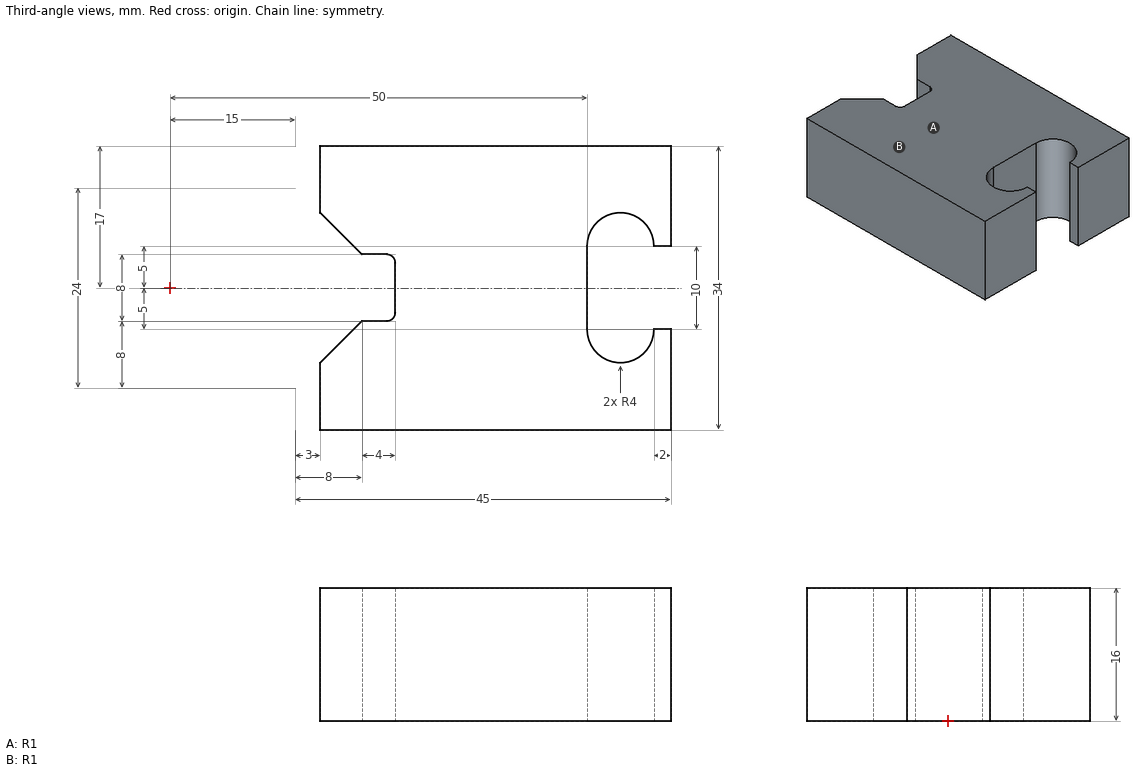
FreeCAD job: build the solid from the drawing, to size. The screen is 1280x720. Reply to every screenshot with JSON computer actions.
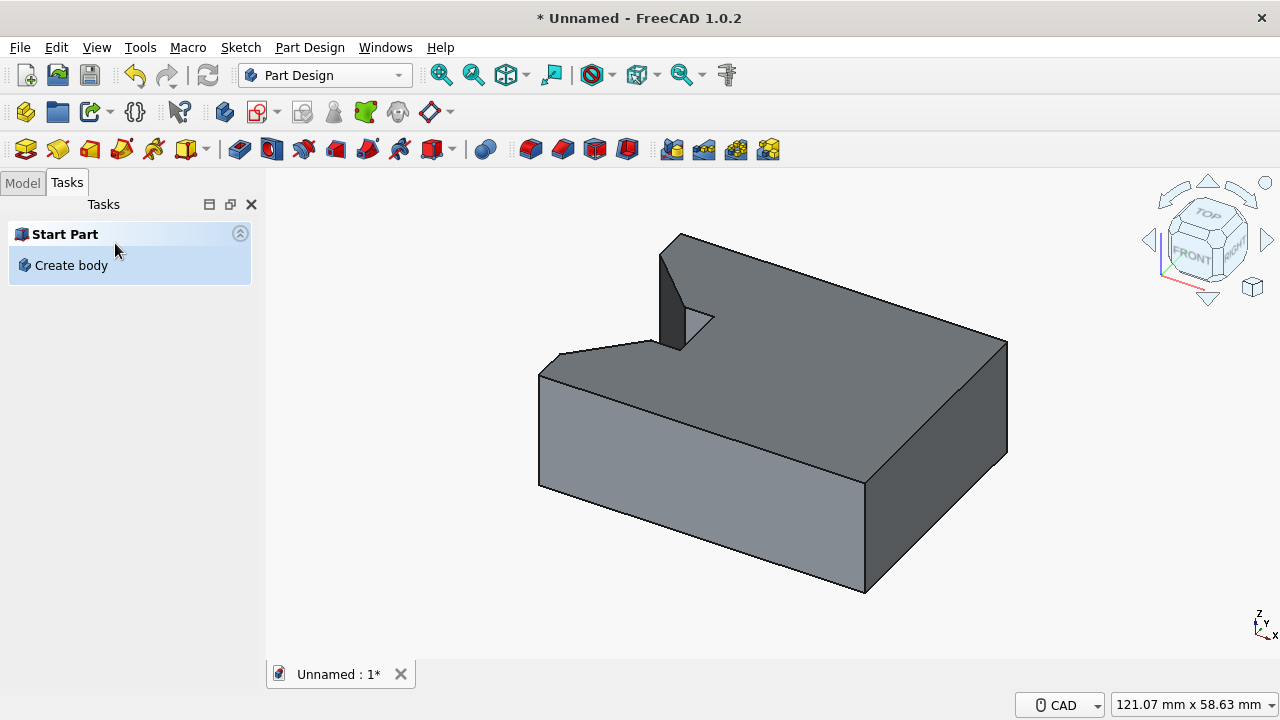
{"action": "key", "text": "0"}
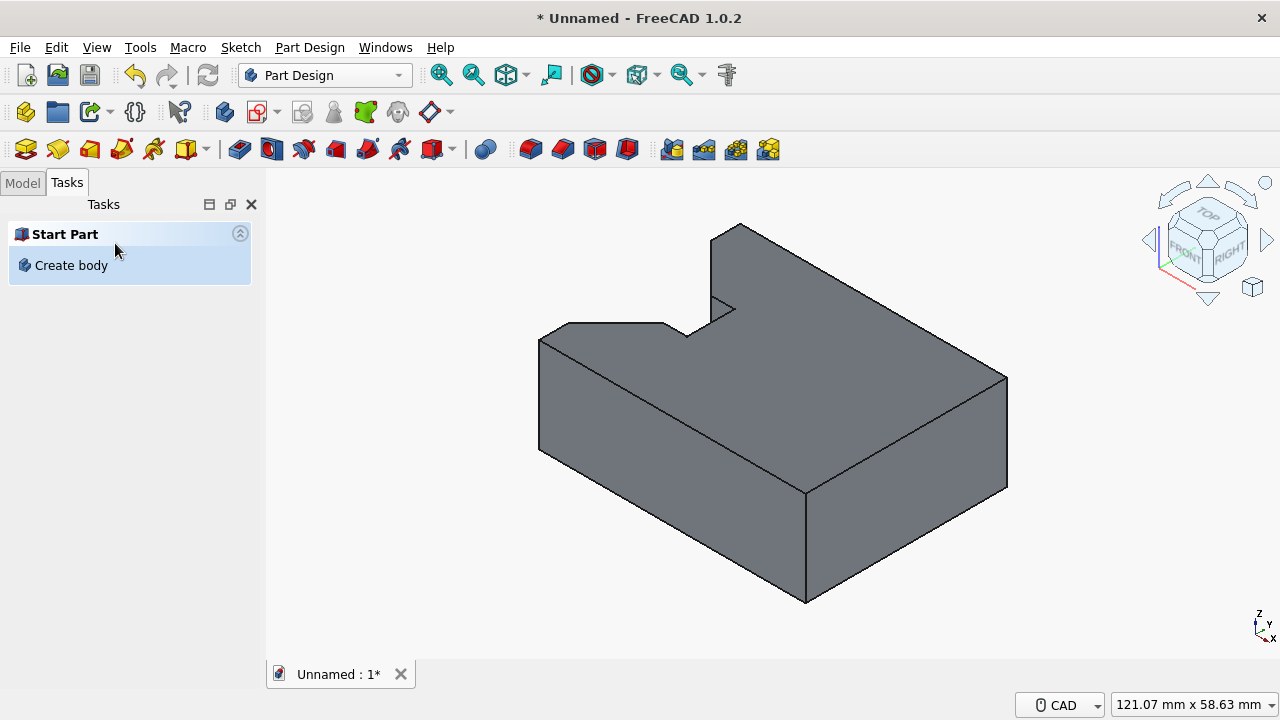
{"action": "key", "text": "2"}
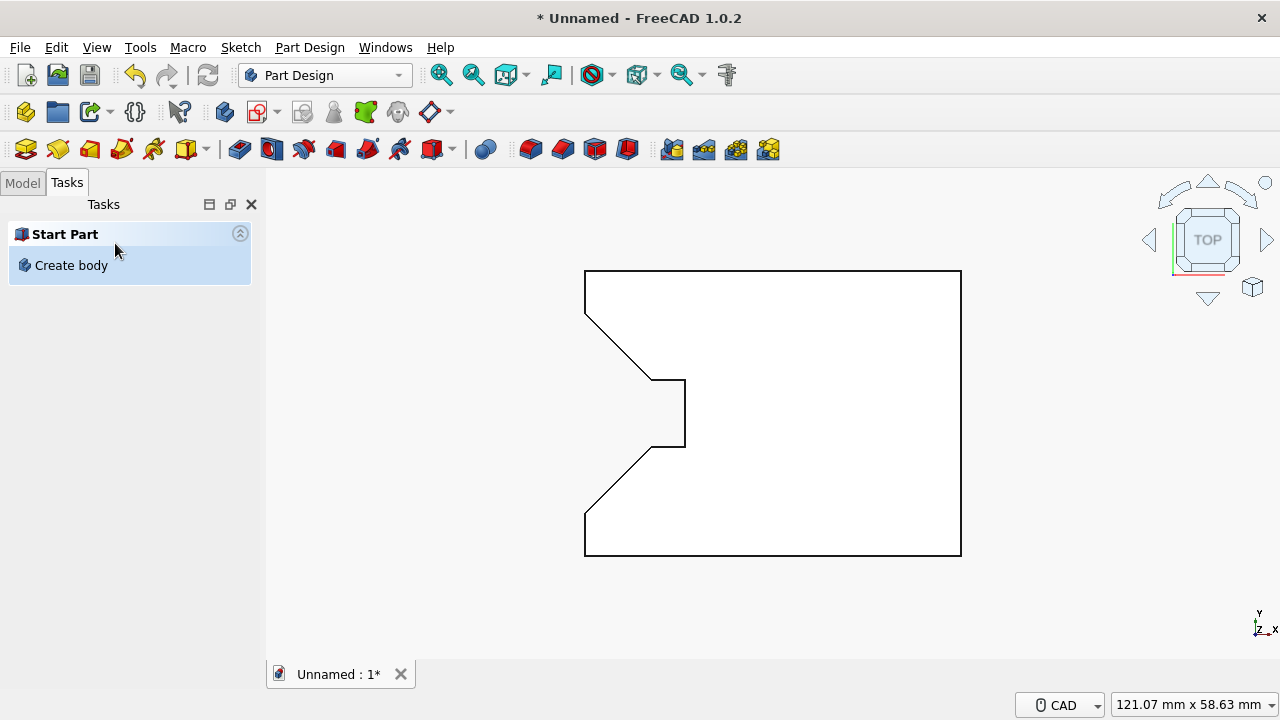
{"action": "key", "text": "1"}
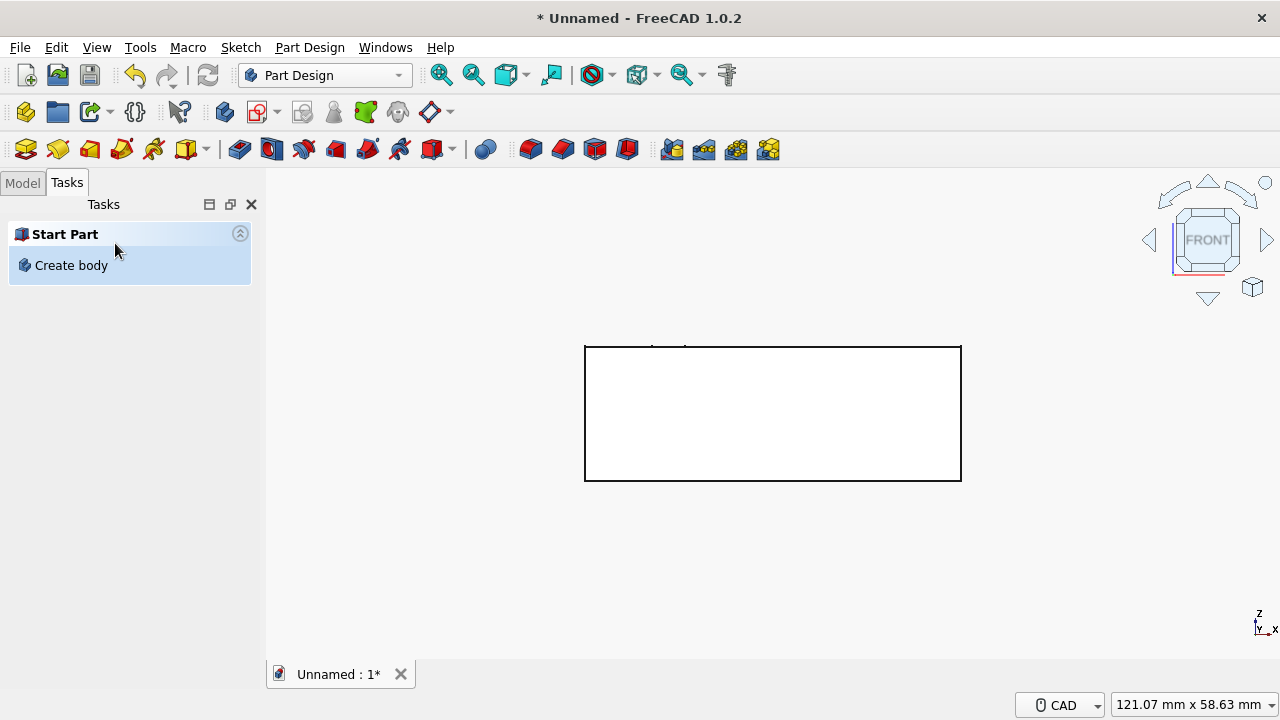
{"action": "left_click", "coordinate": [442, 76]}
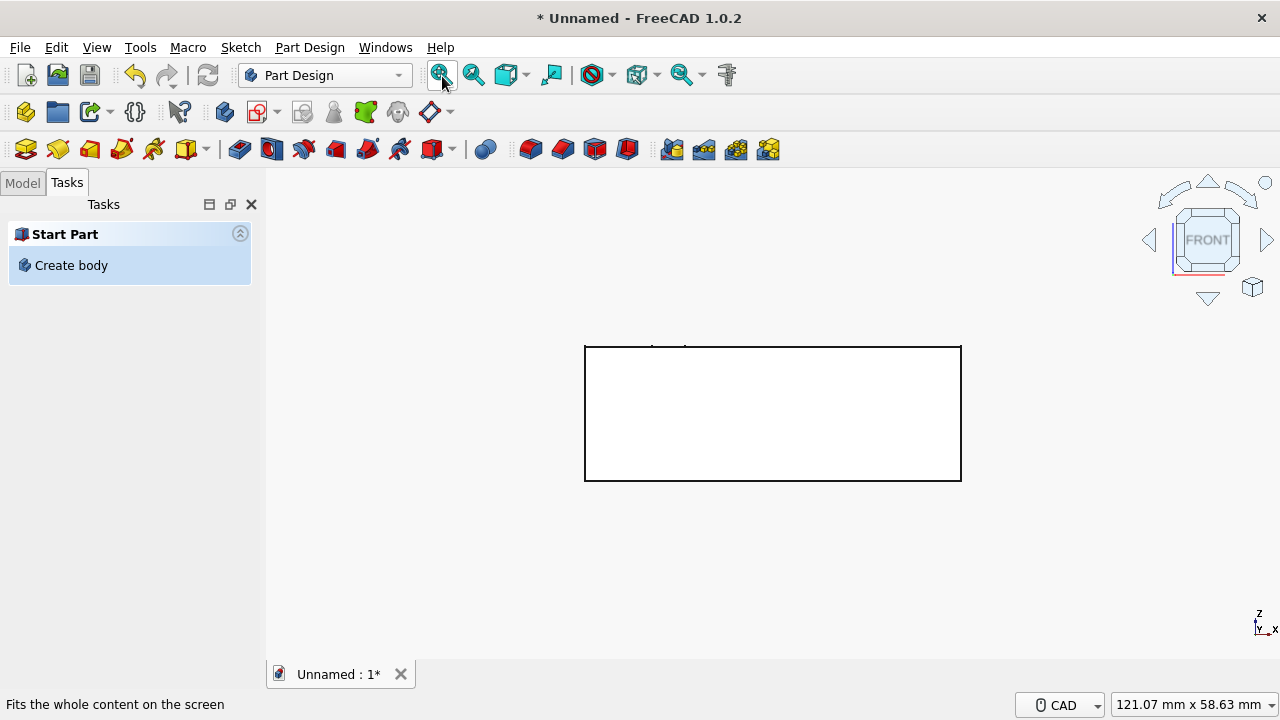
{"action": "key", "text": "3"}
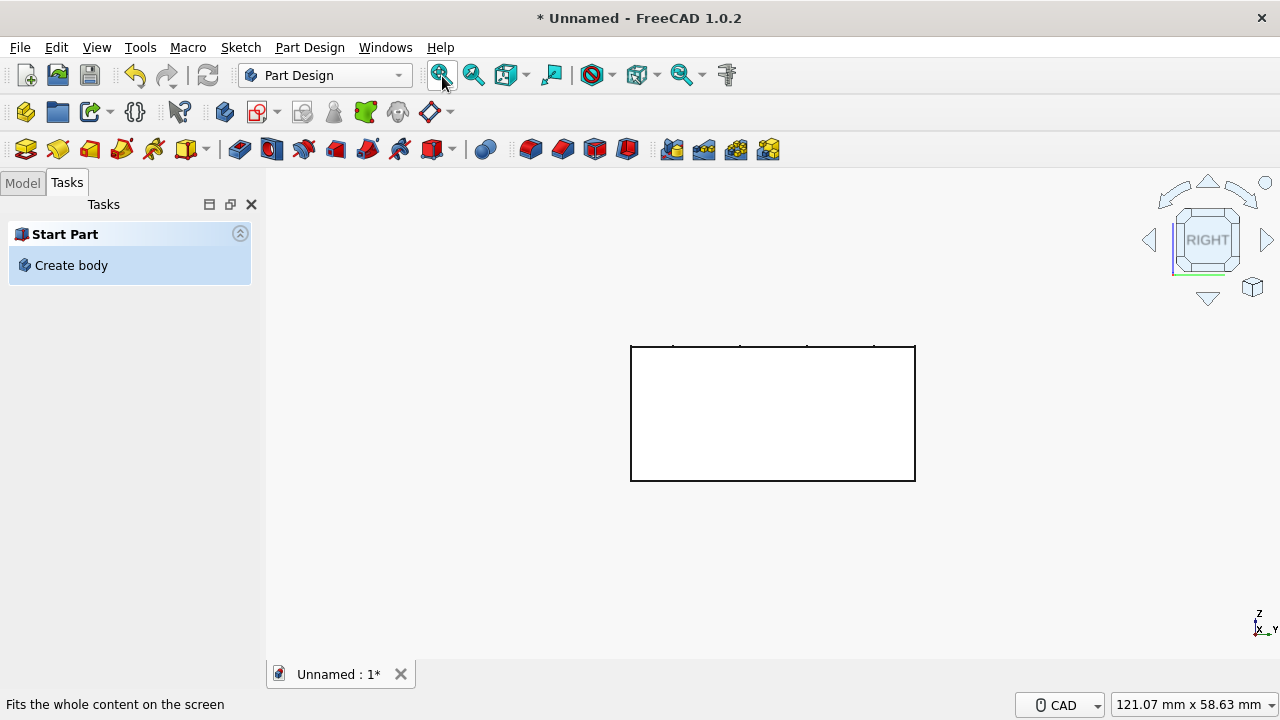
{"action": "left_click", "coordinate": [442, 76]}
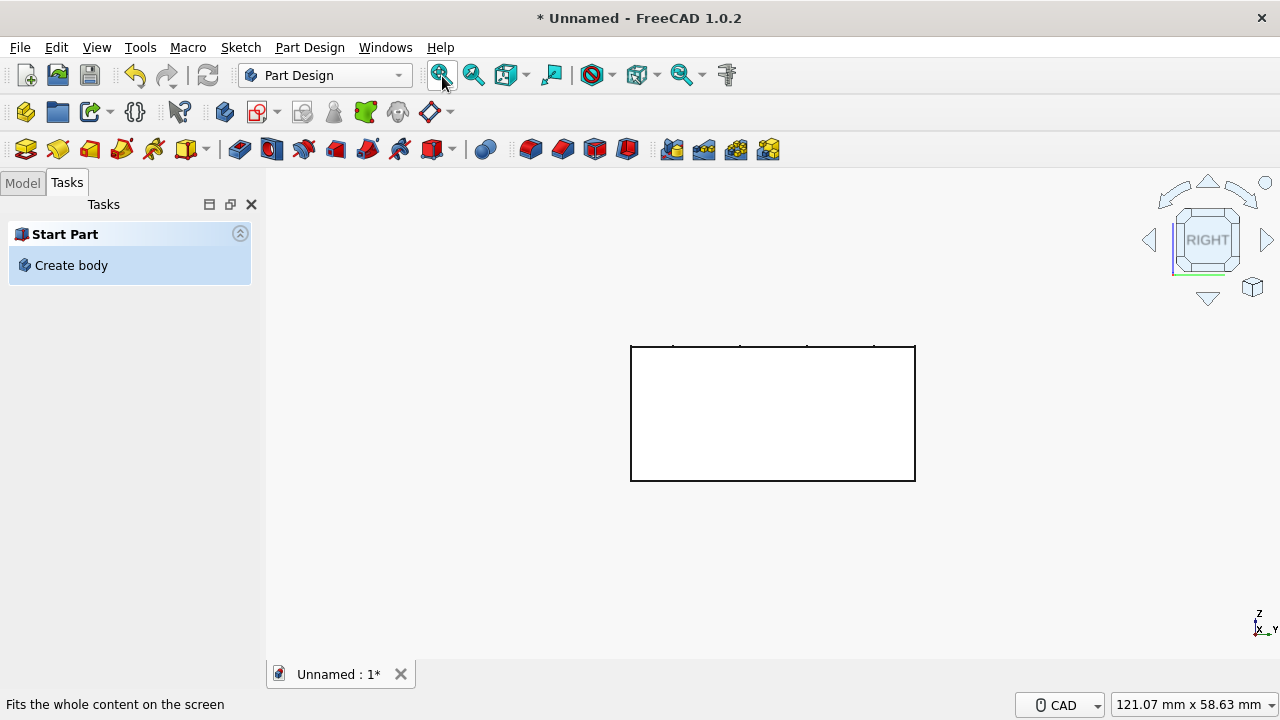
{"action": "key", "text": "5"}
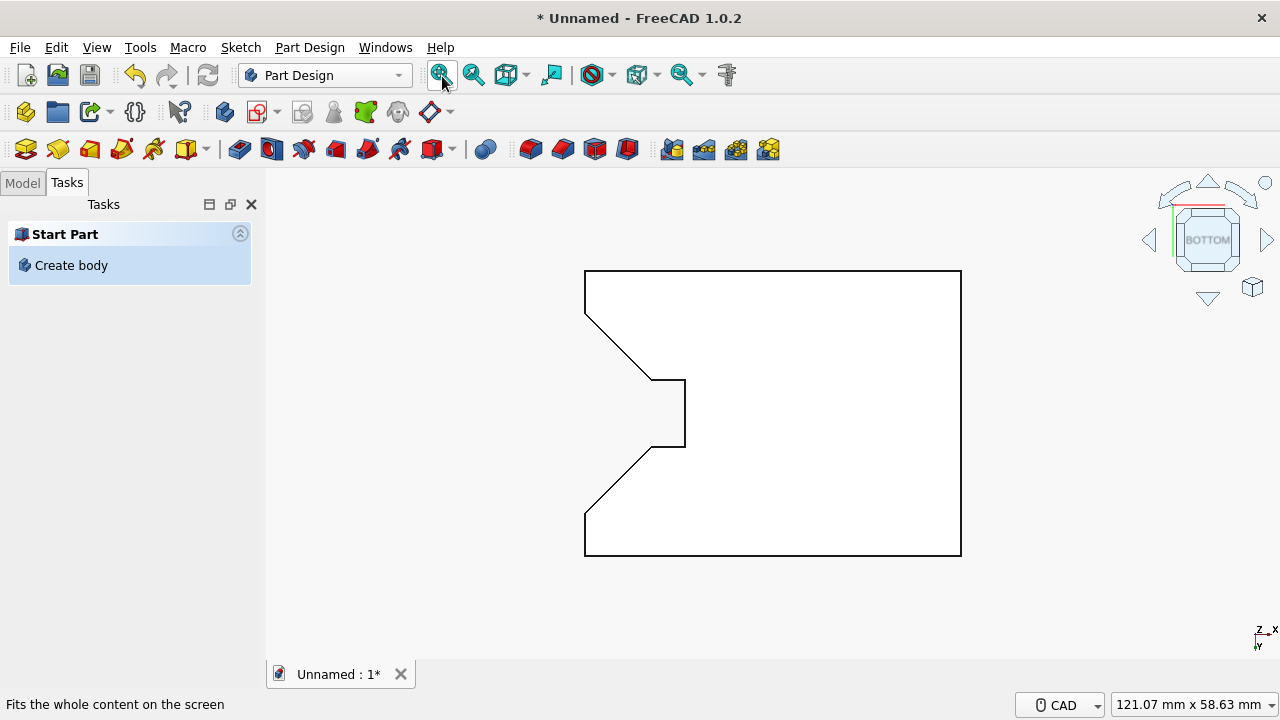
{"action": "key", "text": "4"}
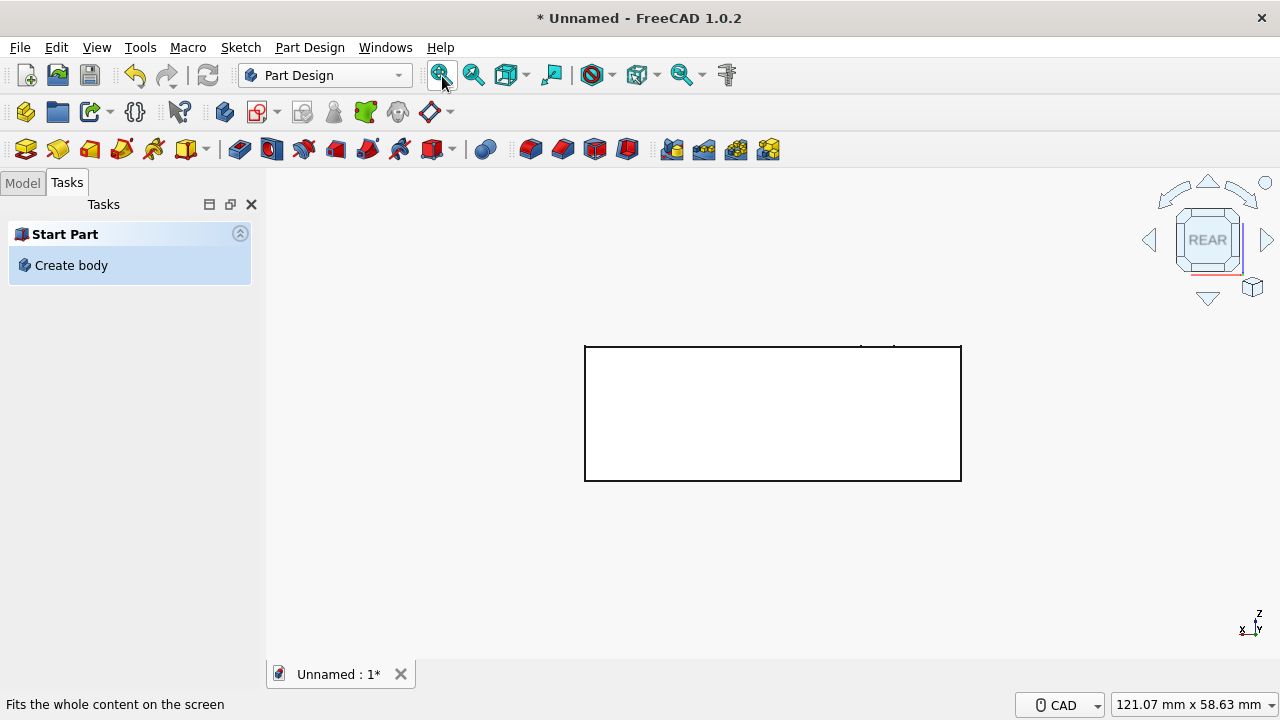
{"action": "left_click", "coordinate": [442, 76]}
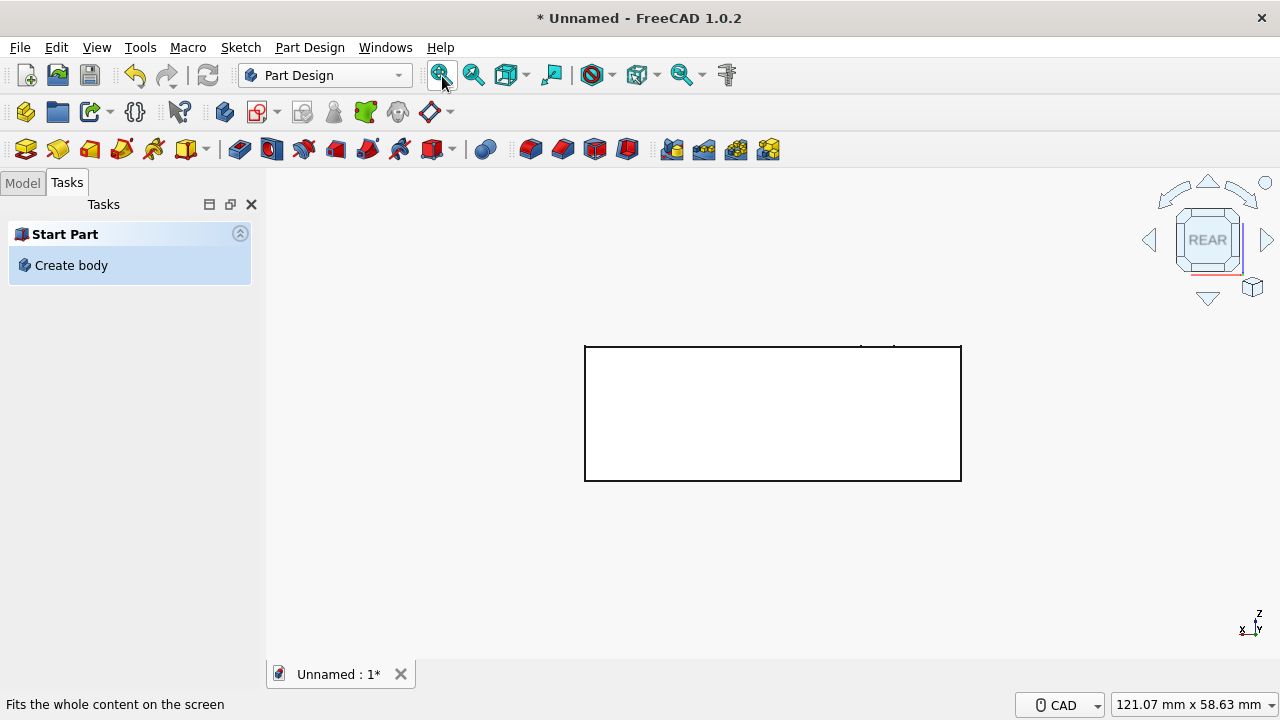
{"action": "key", "text": "6"}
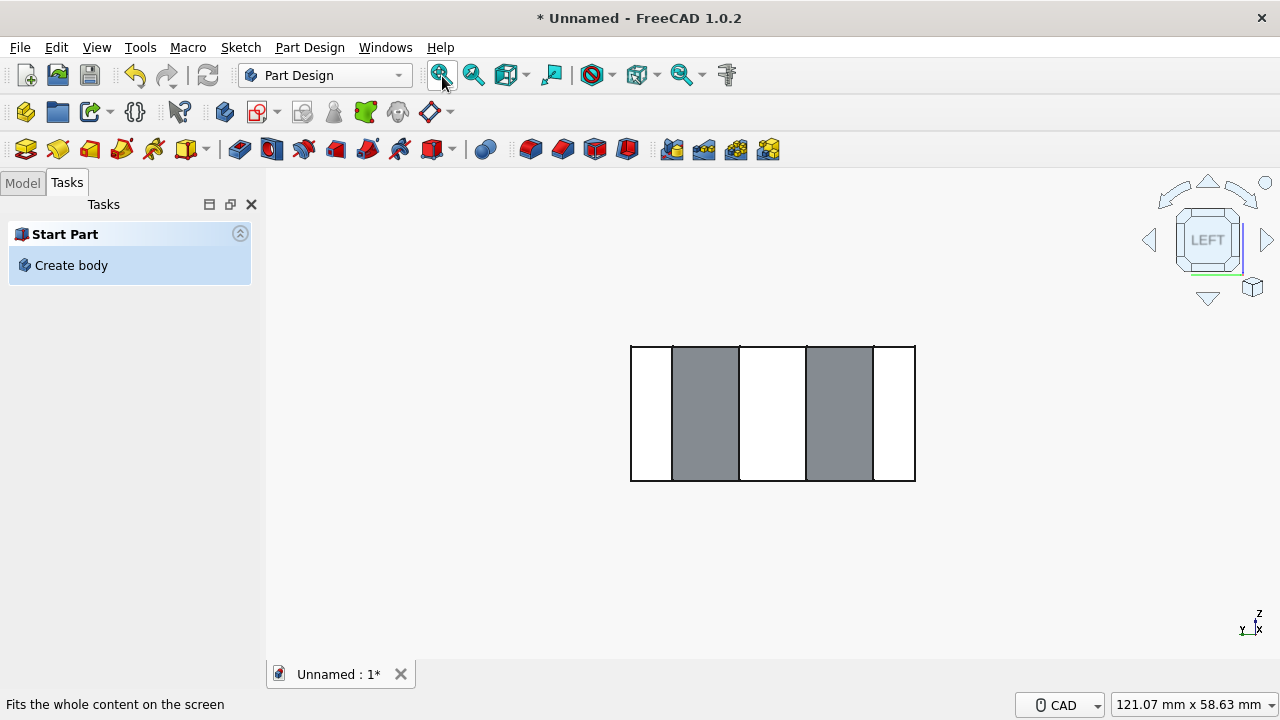
{"action": "left_click", "coordinate": [442, 76]}